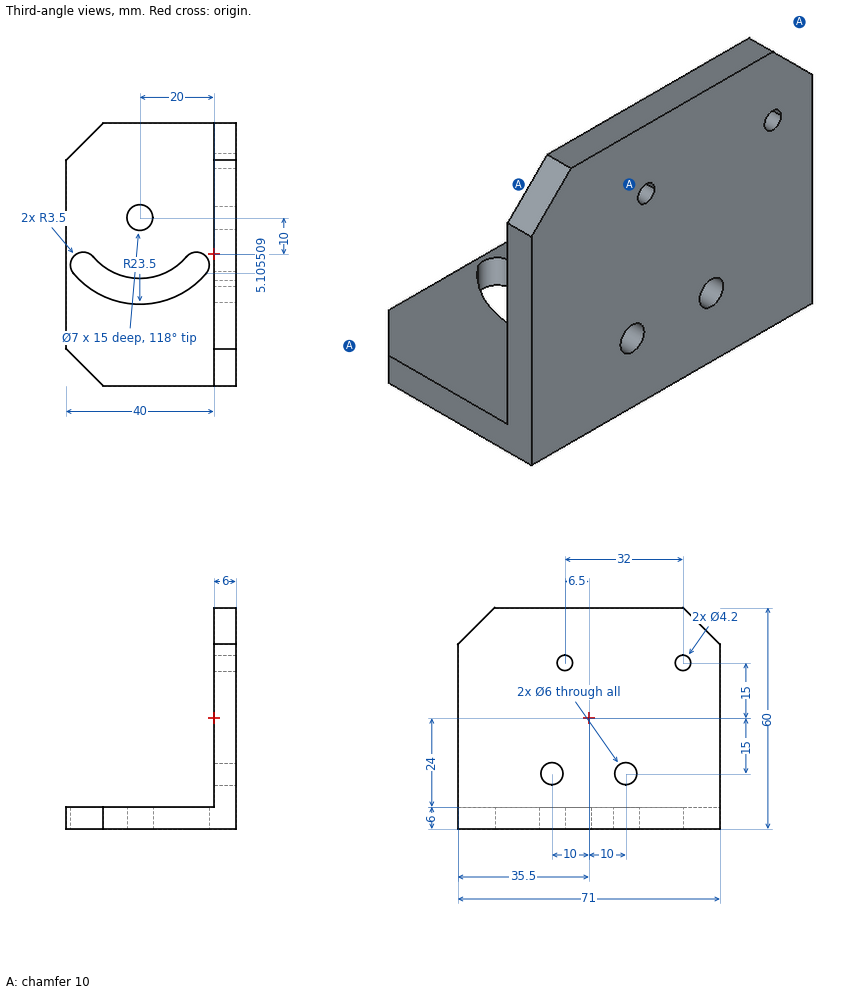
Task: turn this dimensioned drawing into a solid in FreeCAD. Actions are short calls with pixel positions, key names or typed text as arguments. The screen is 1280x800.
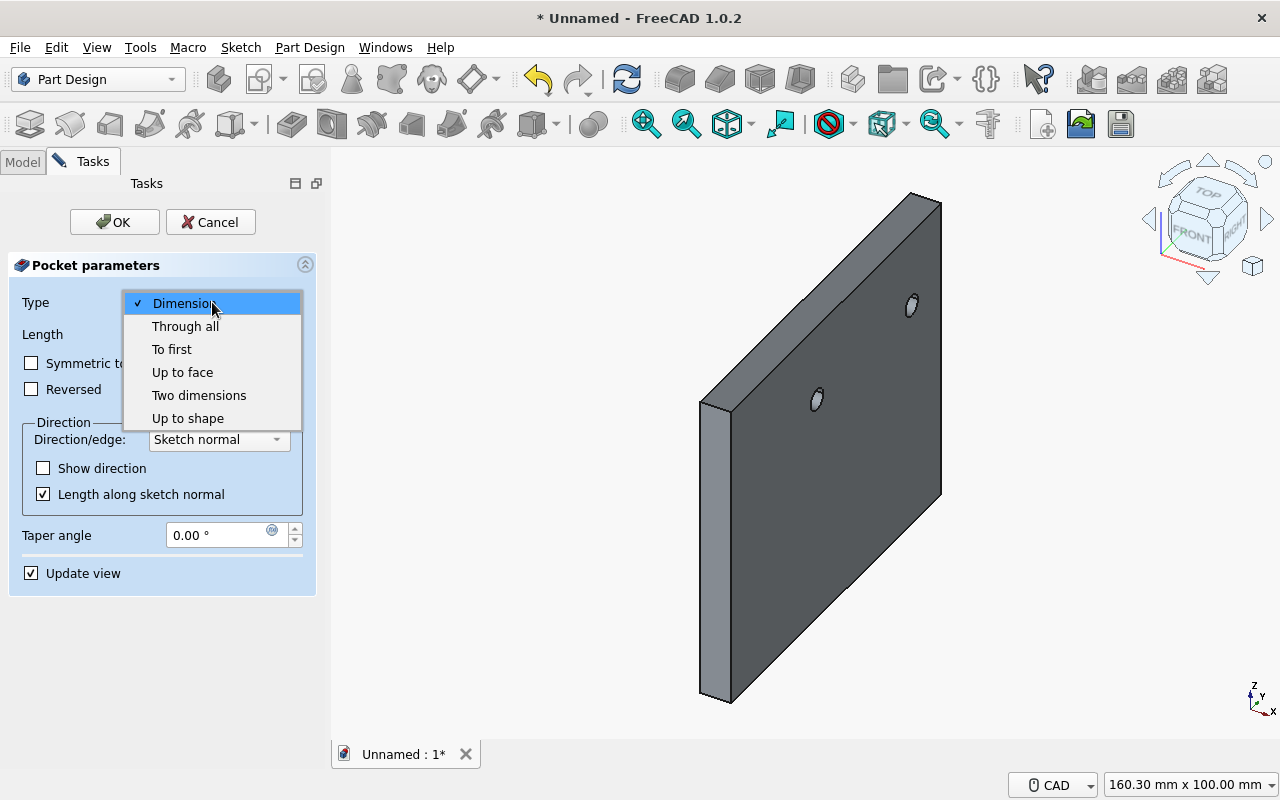
click(212, 326)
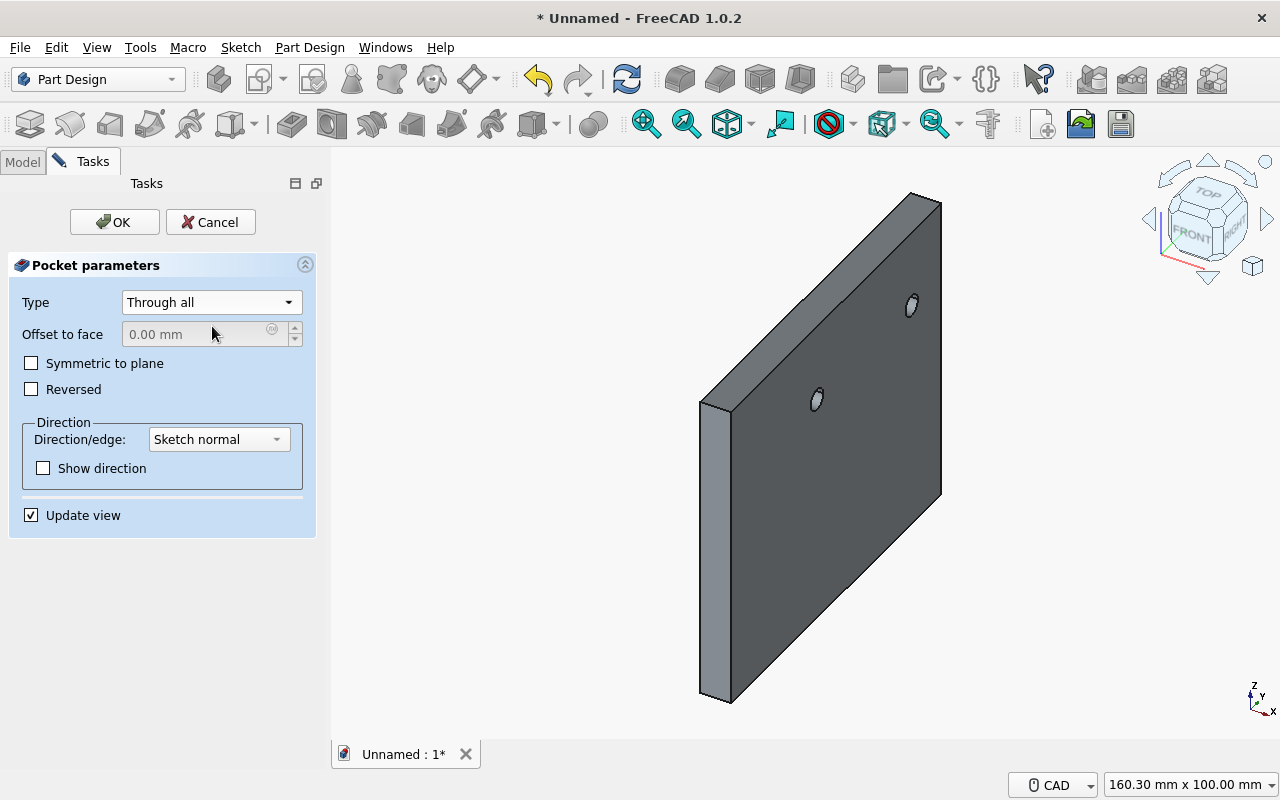
click(115, 222)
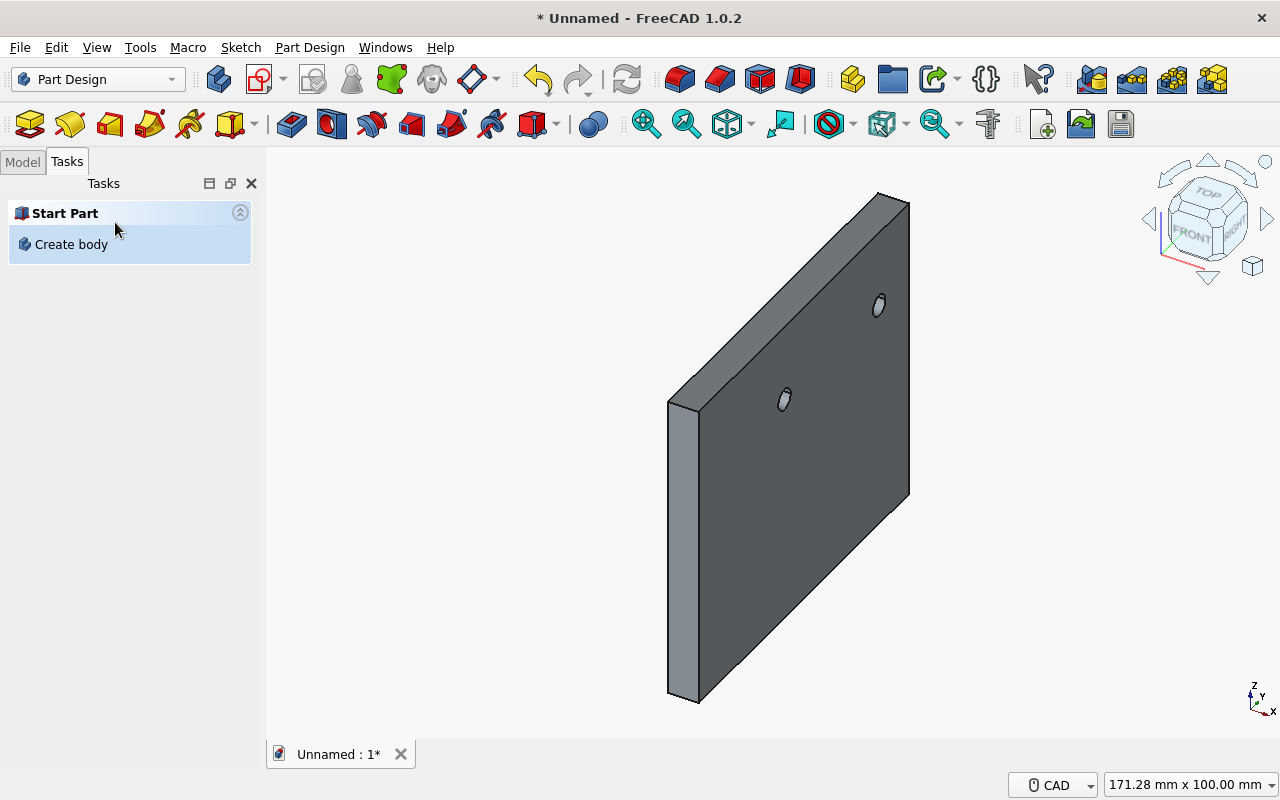
key(6)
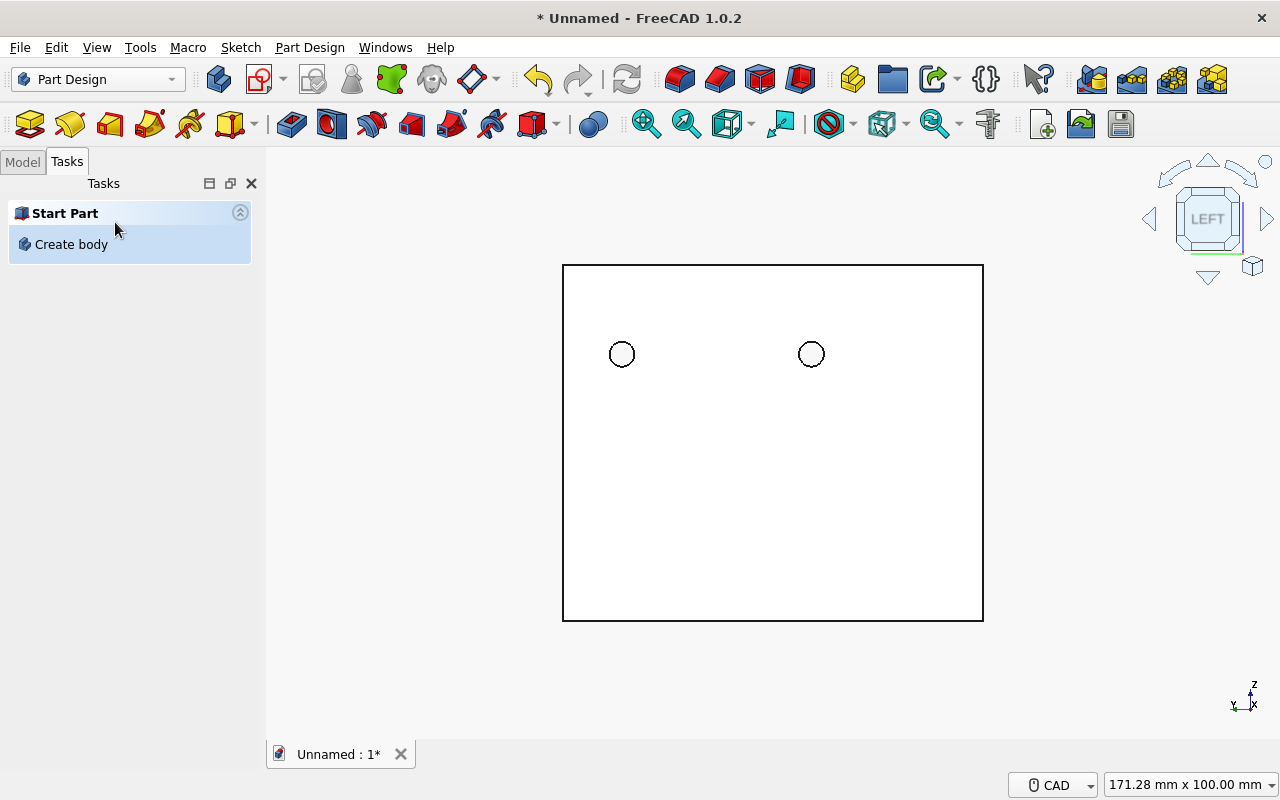
click(713, 493)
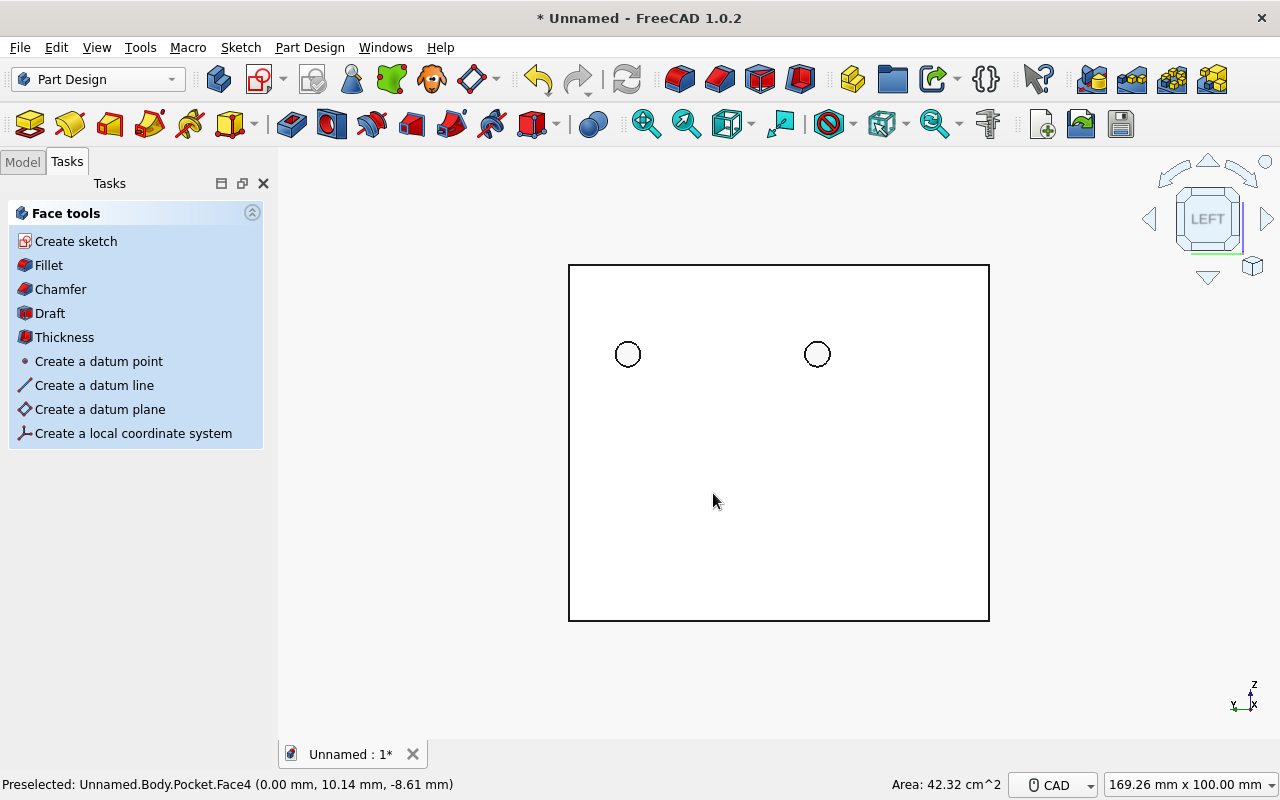
click(260, 80)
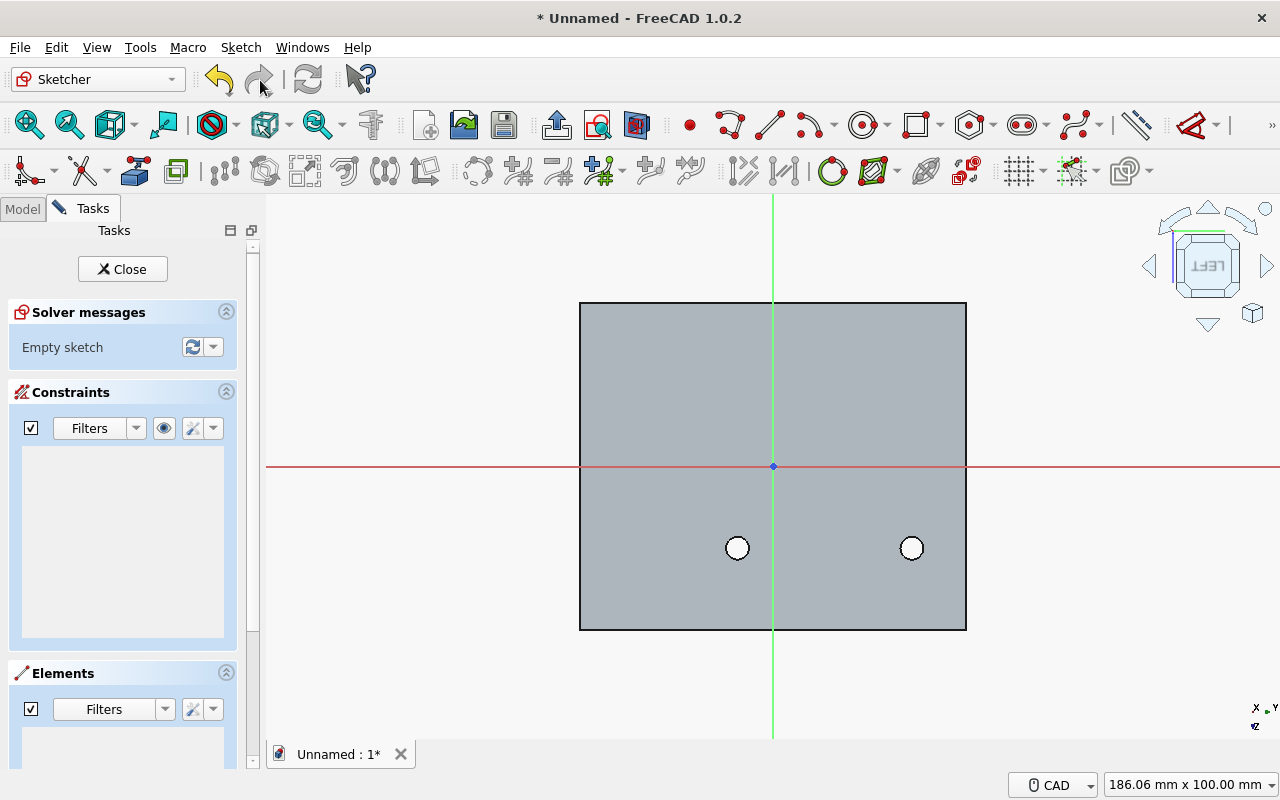
scroll(803, 396, up, 6)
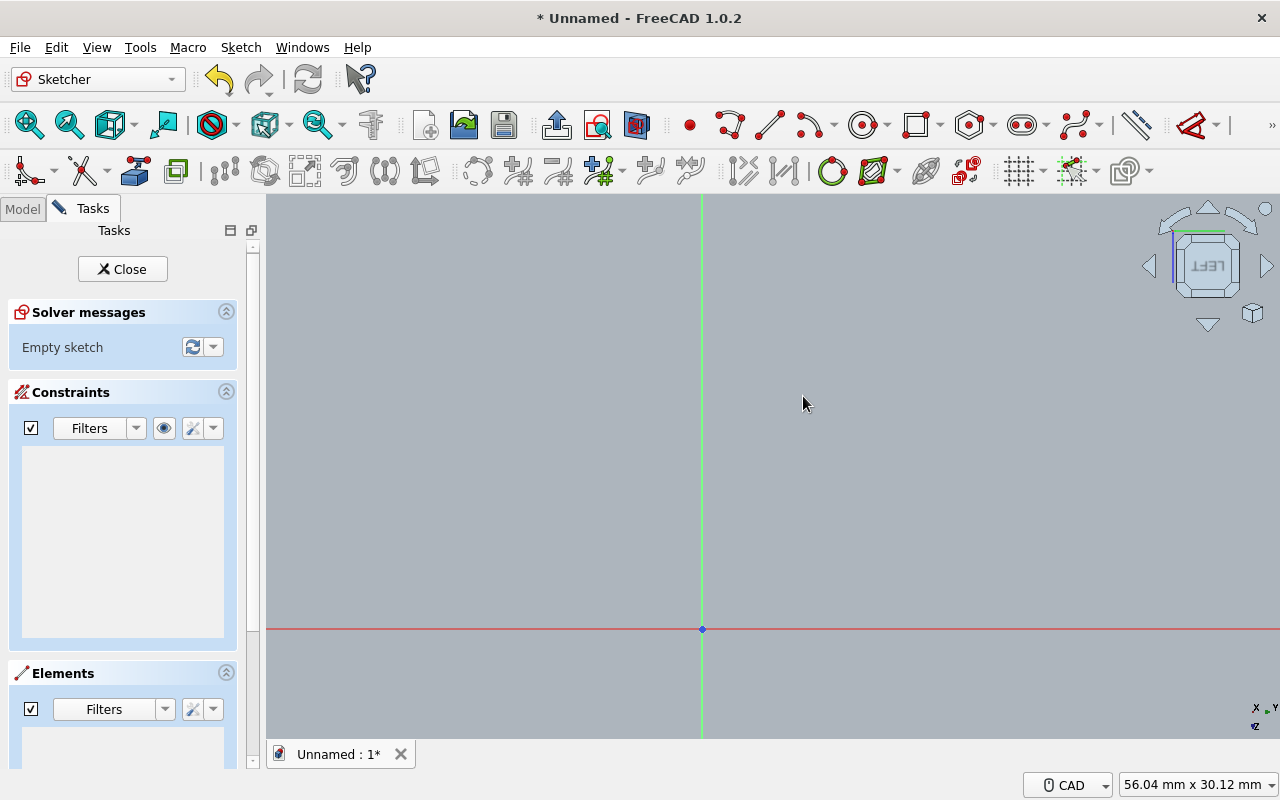
click(864, 126)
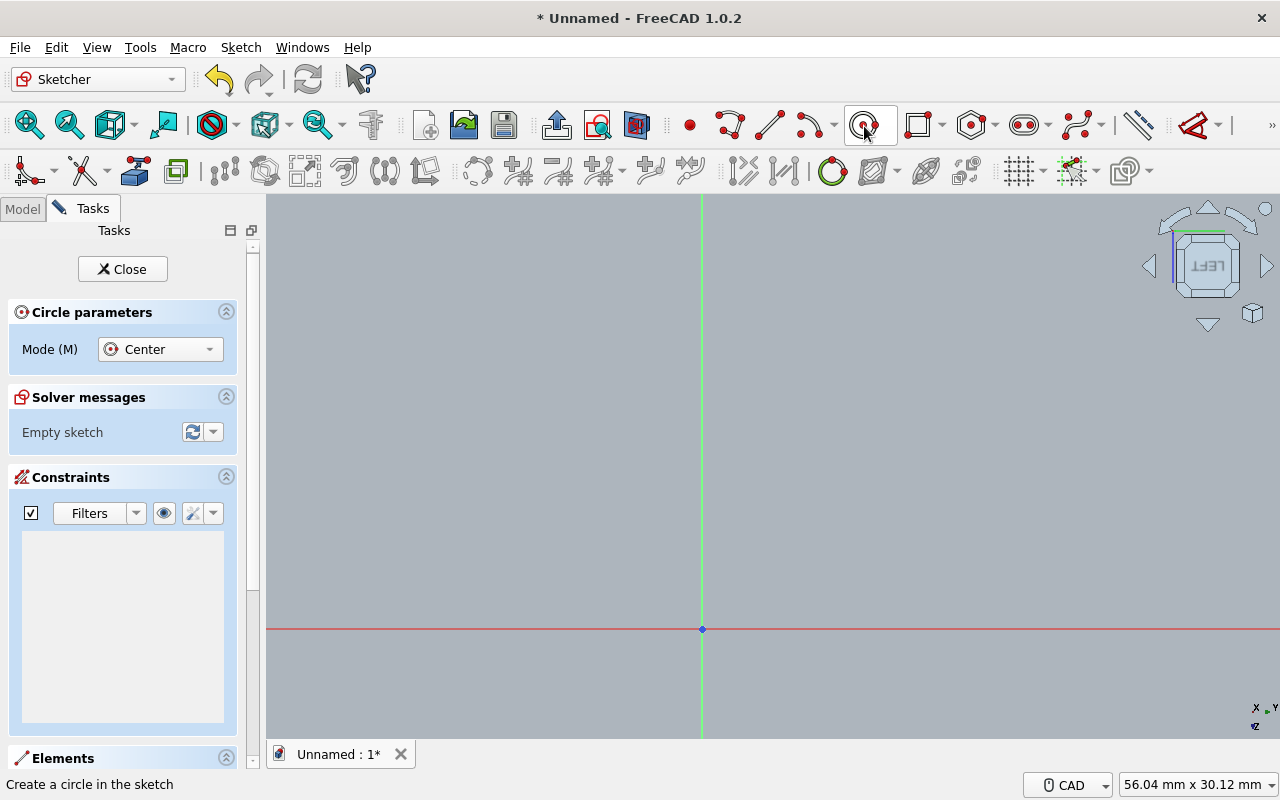
click(883, 358)
click(921, 319)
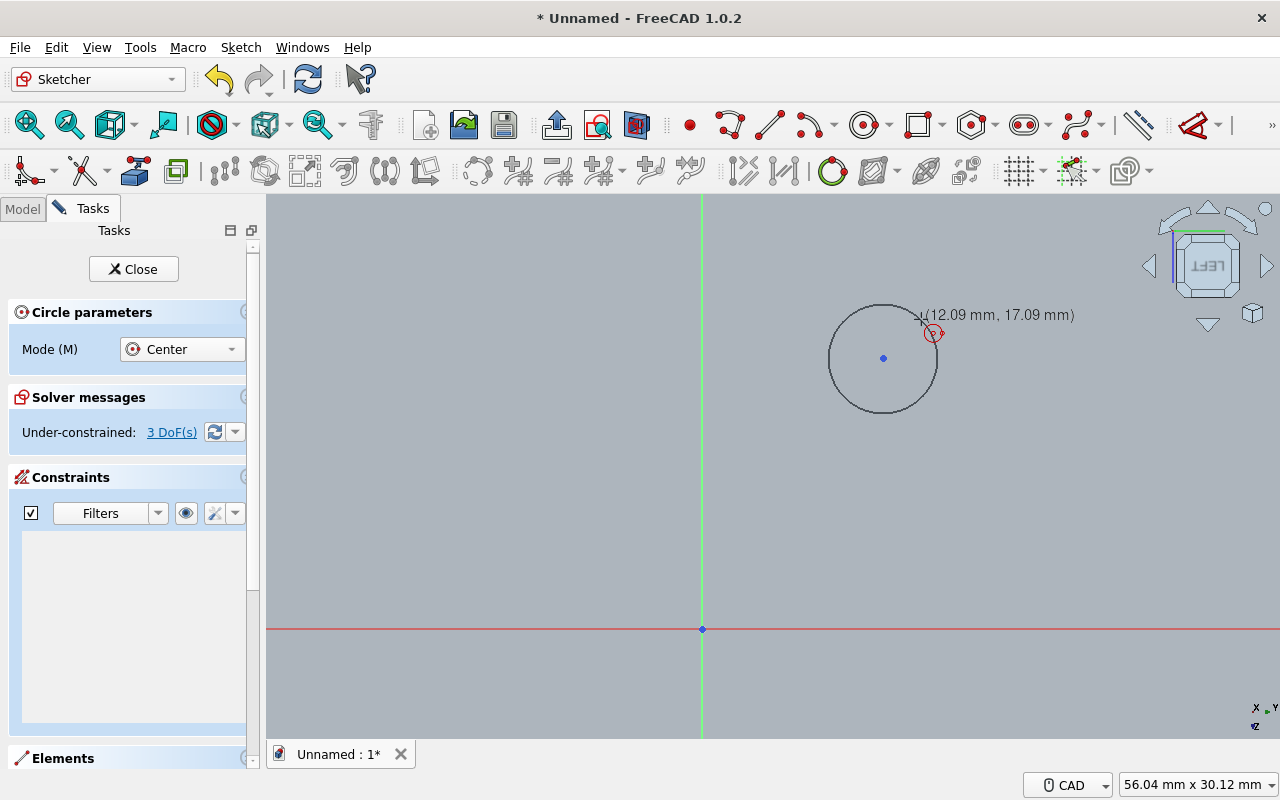
click(521, 358)
click(560, 319)
key(Escape)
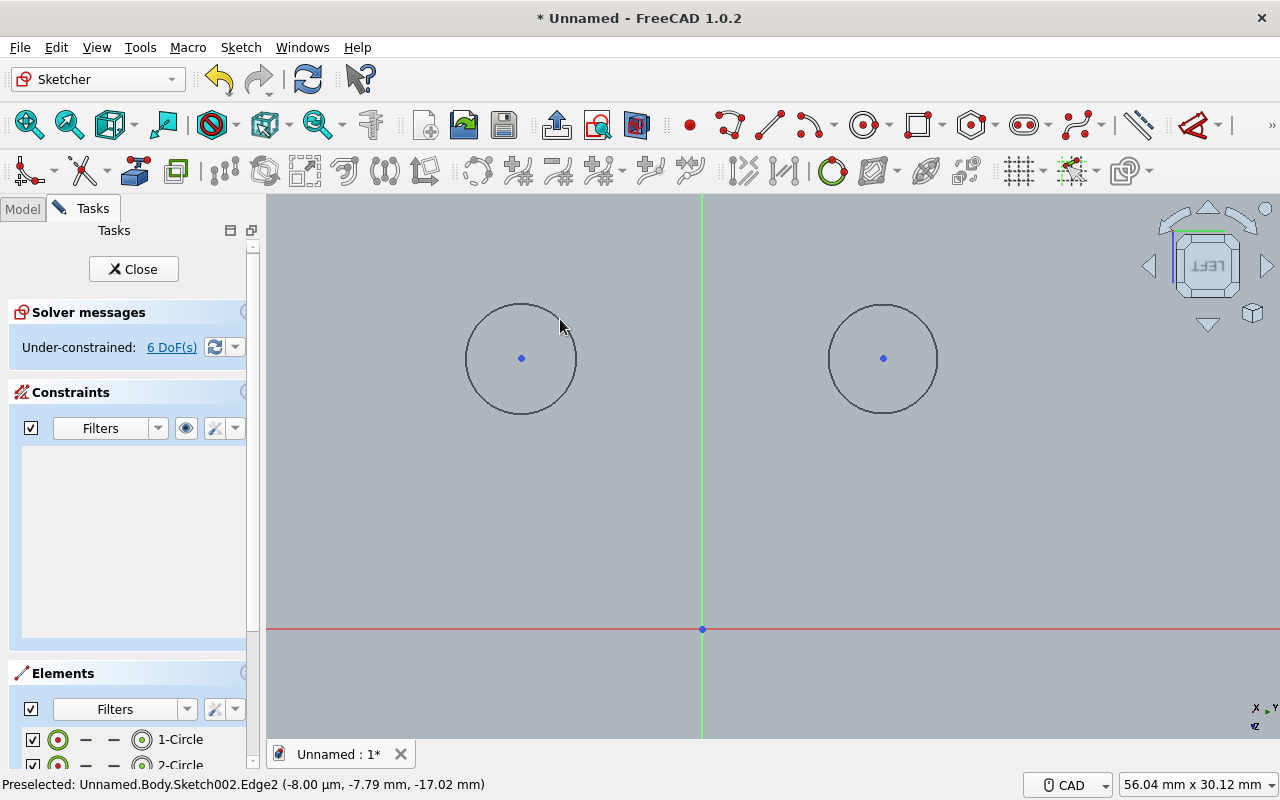
click(921, 320)